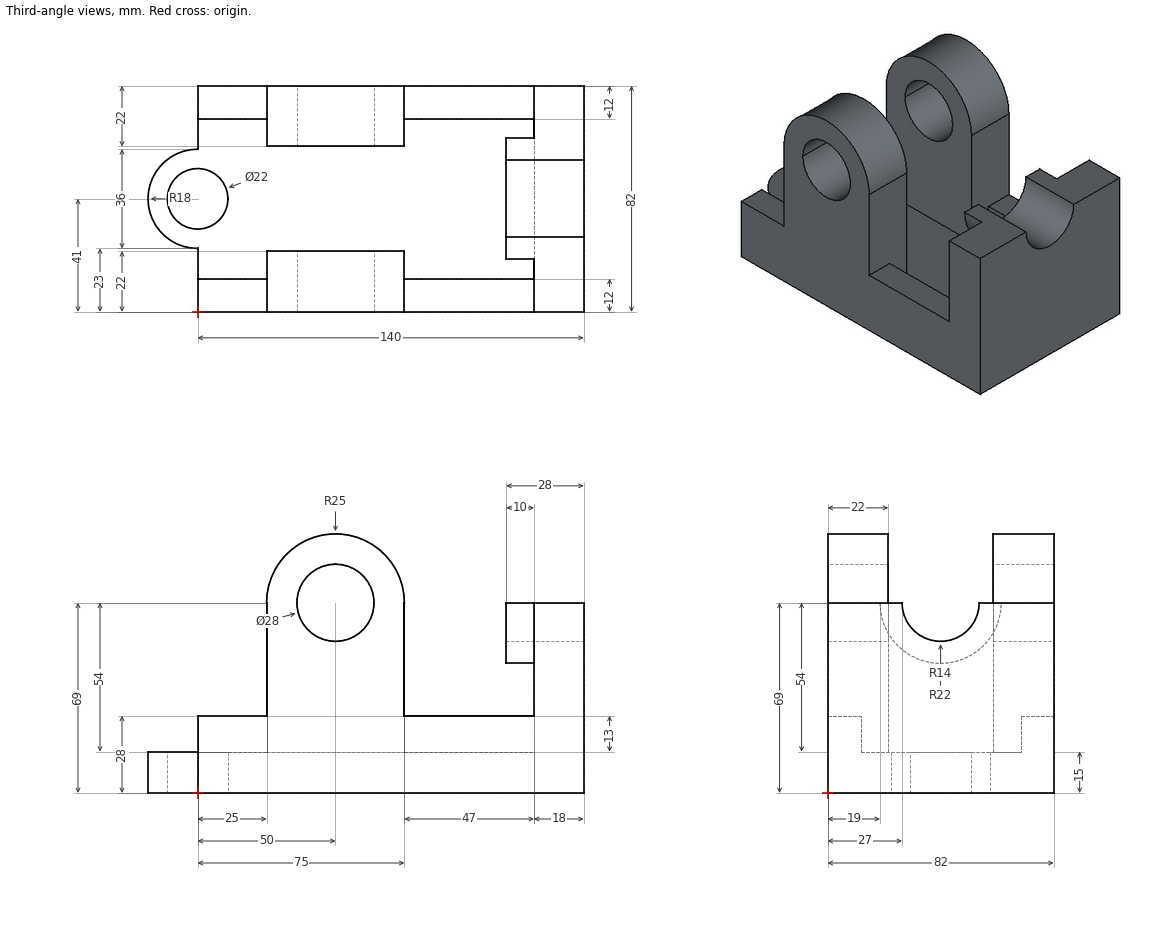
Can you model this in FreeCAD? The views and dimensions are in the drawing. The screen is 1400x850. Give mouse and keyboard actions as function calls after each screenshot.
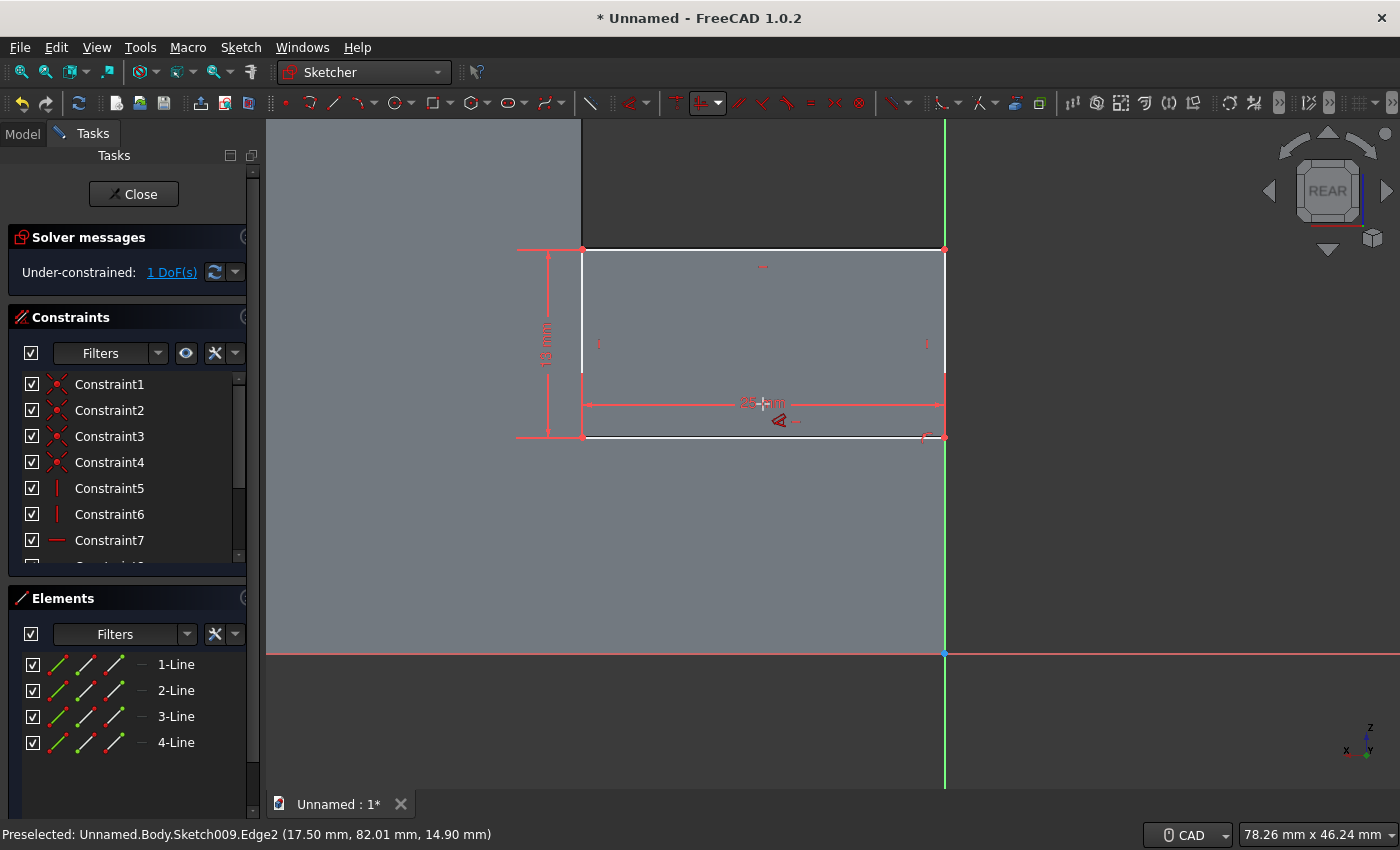
click(582, 250)
click(979, 452)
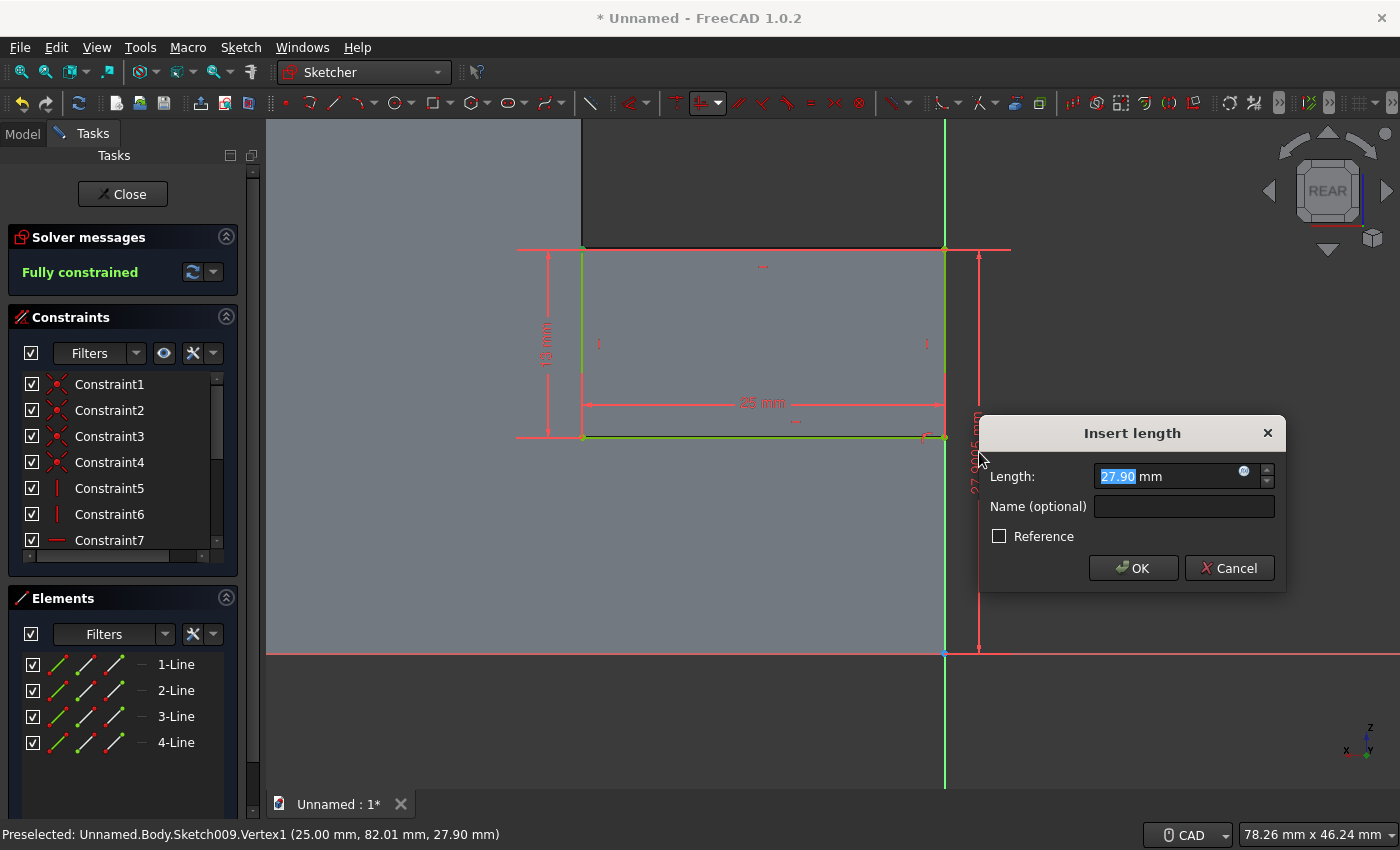
text(28)
key(Return)
key(Escape)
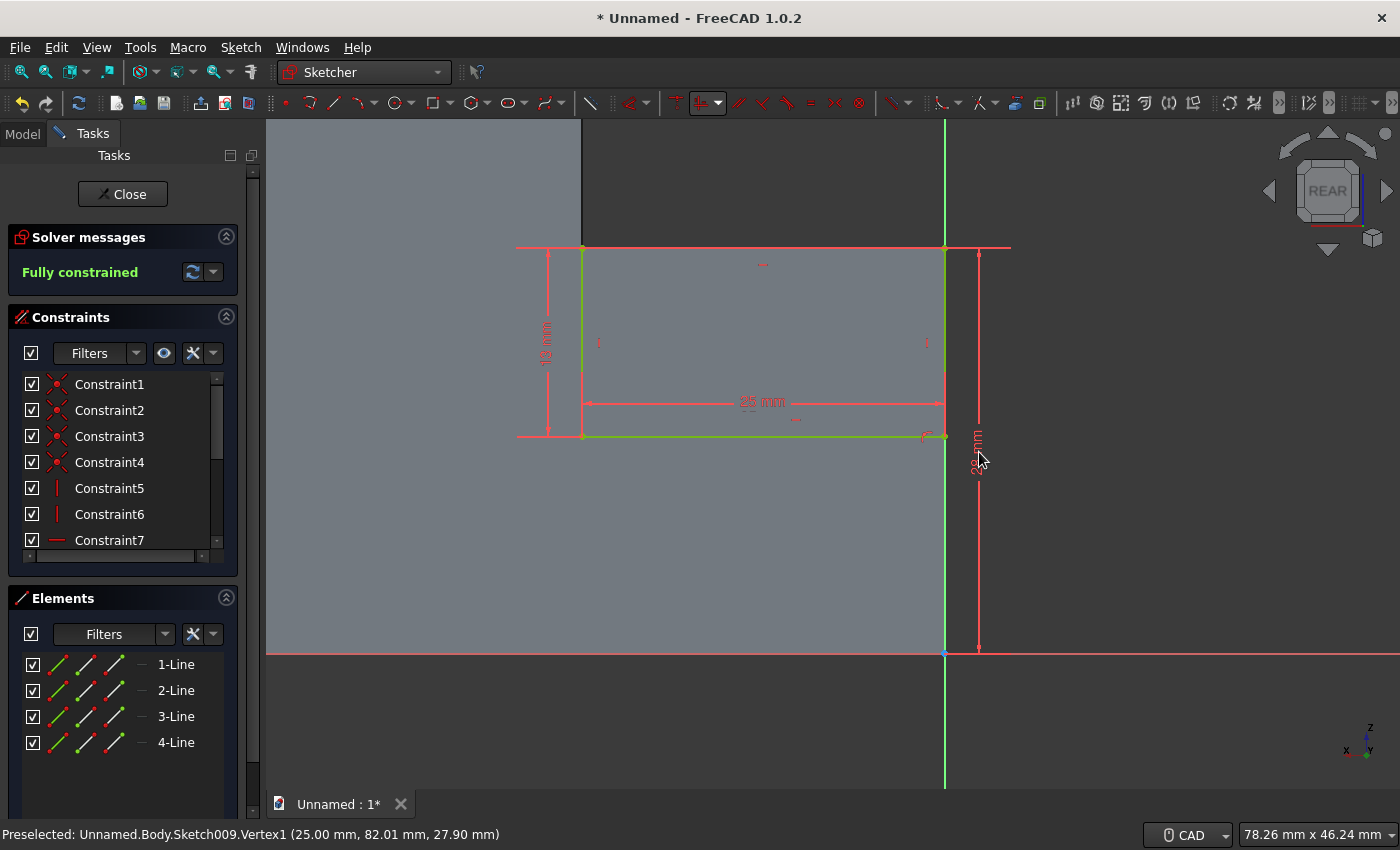
click(123, 194)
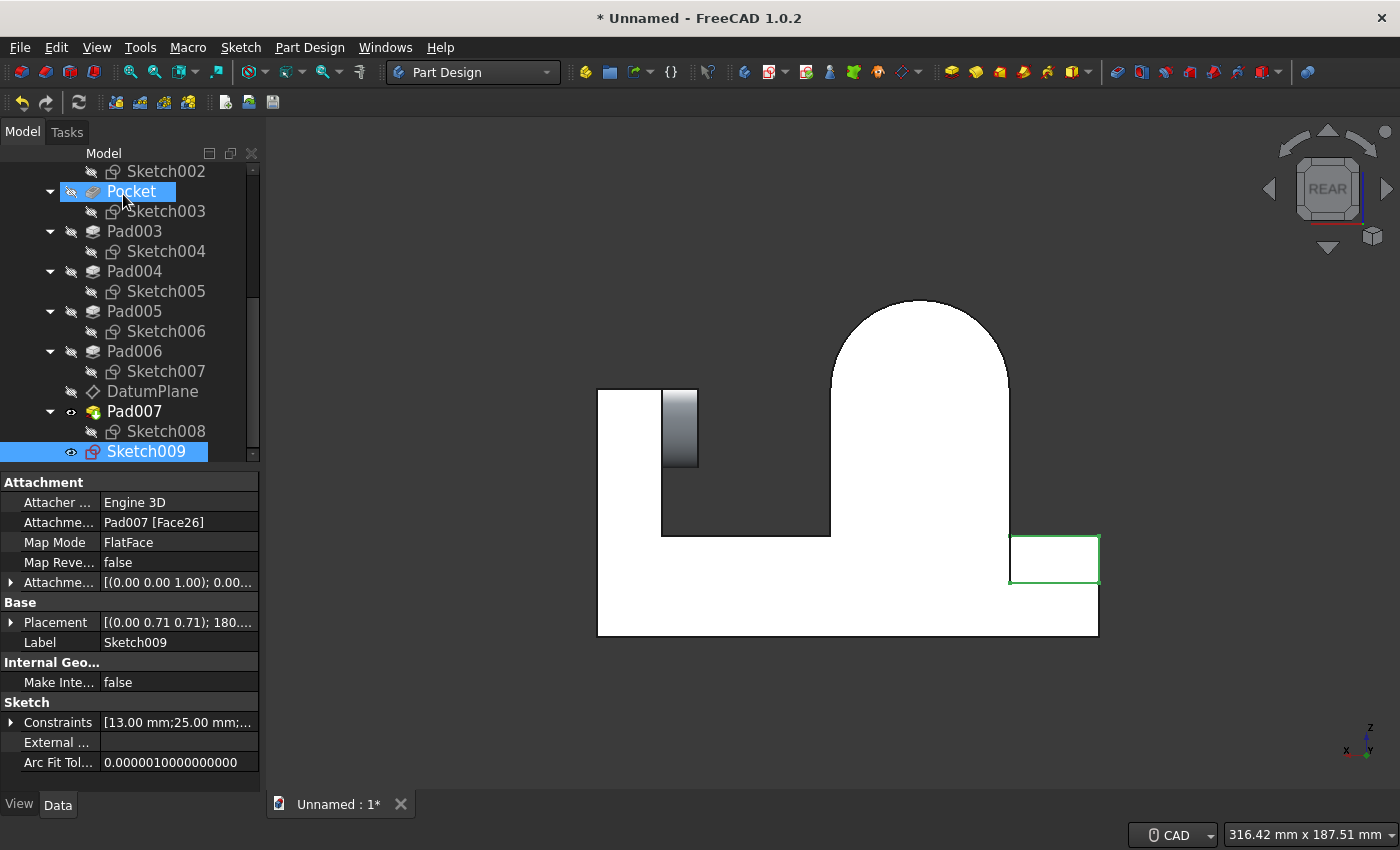
click(952, 72)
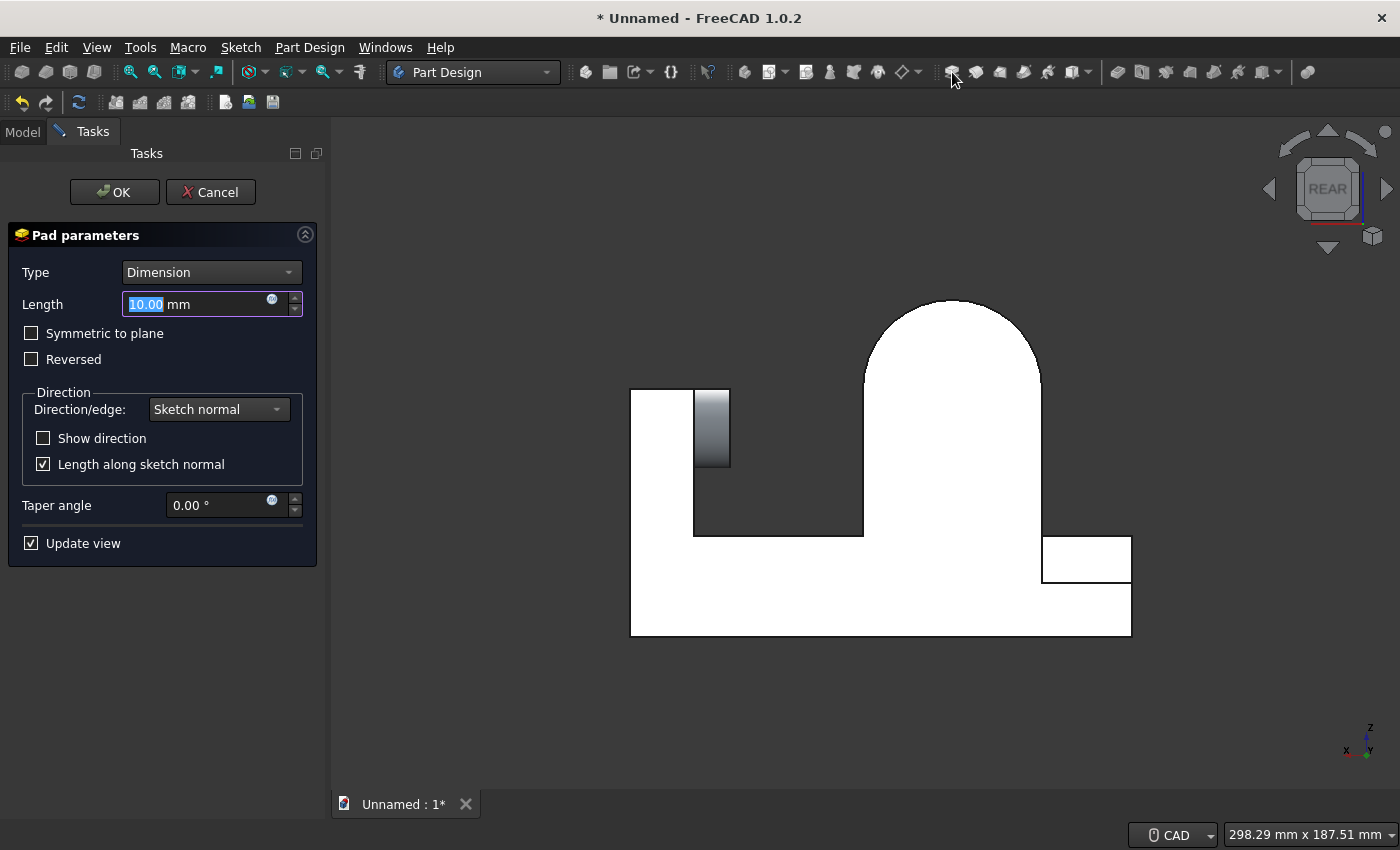
text(12)
key(Tab)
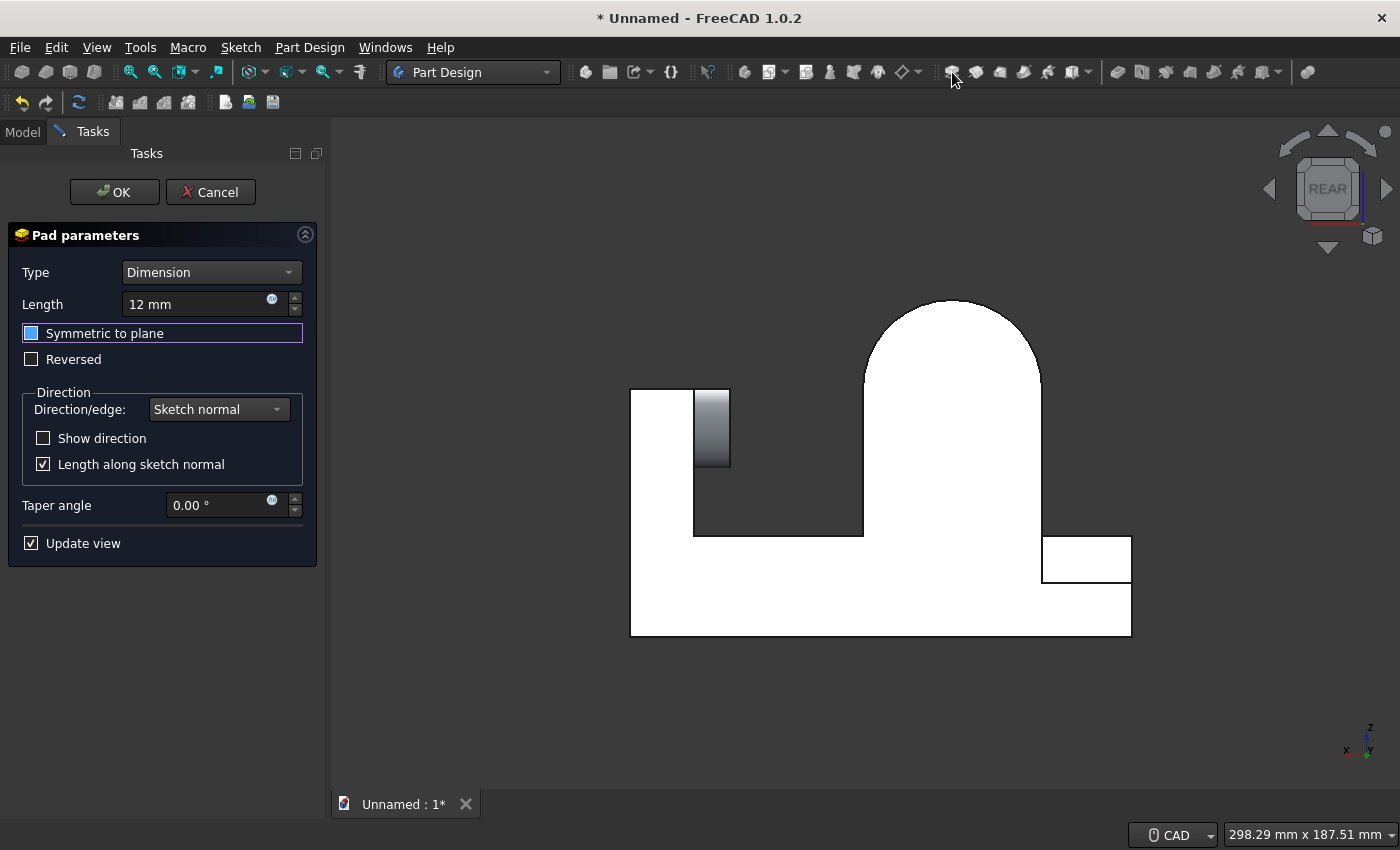
click(30, 359)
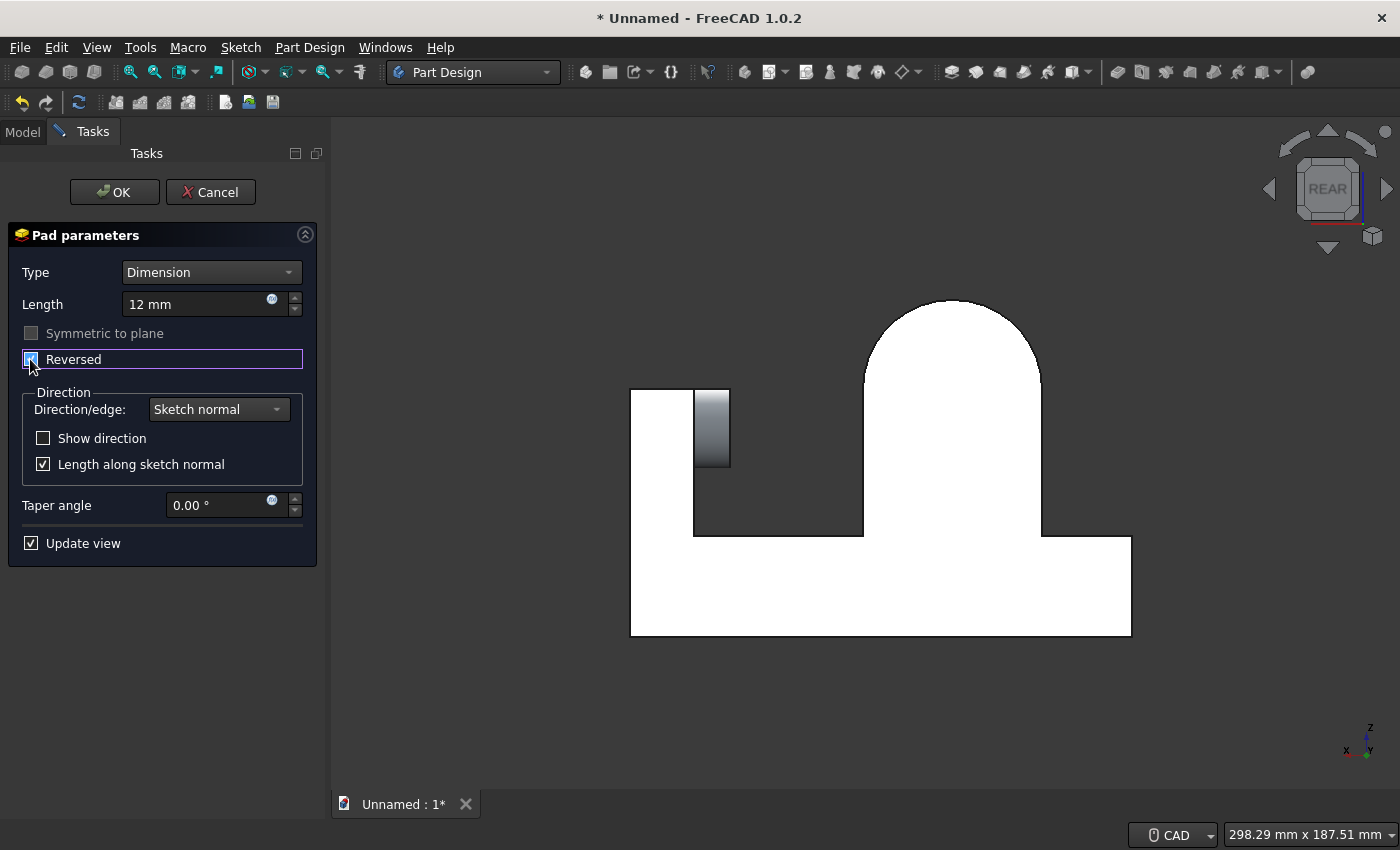
click(115, 192)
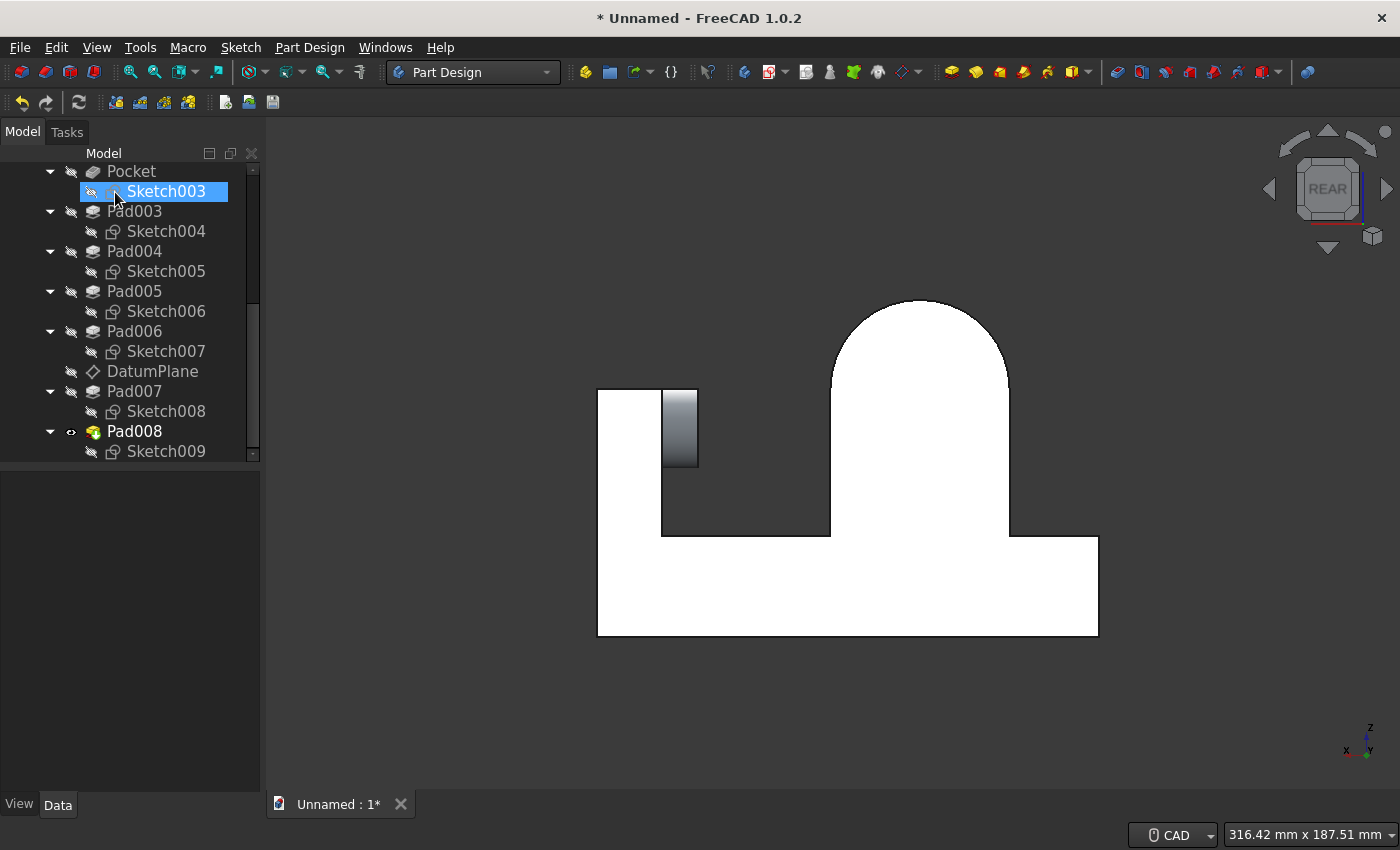
key(0)